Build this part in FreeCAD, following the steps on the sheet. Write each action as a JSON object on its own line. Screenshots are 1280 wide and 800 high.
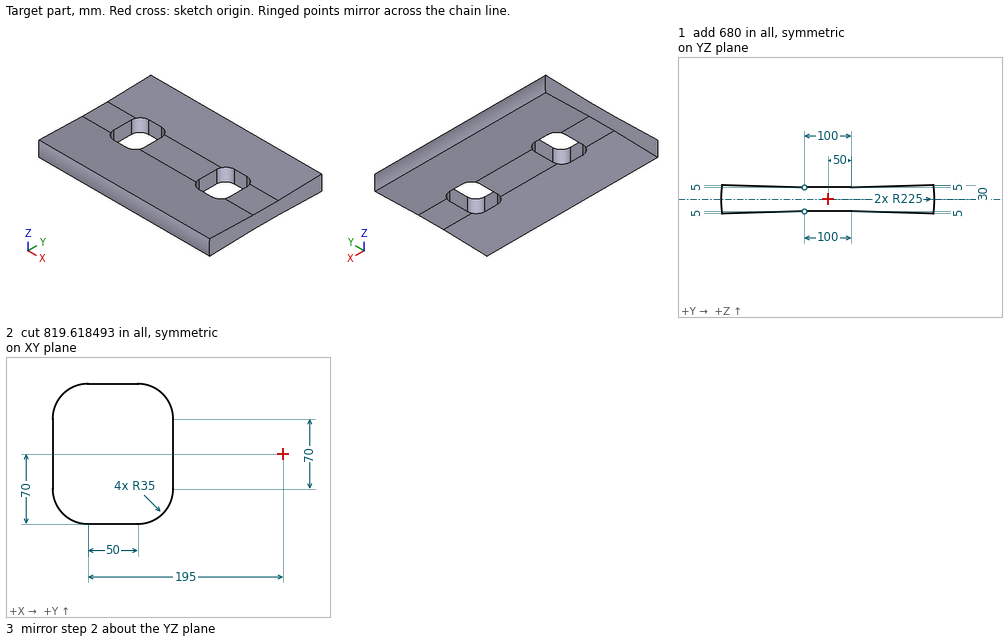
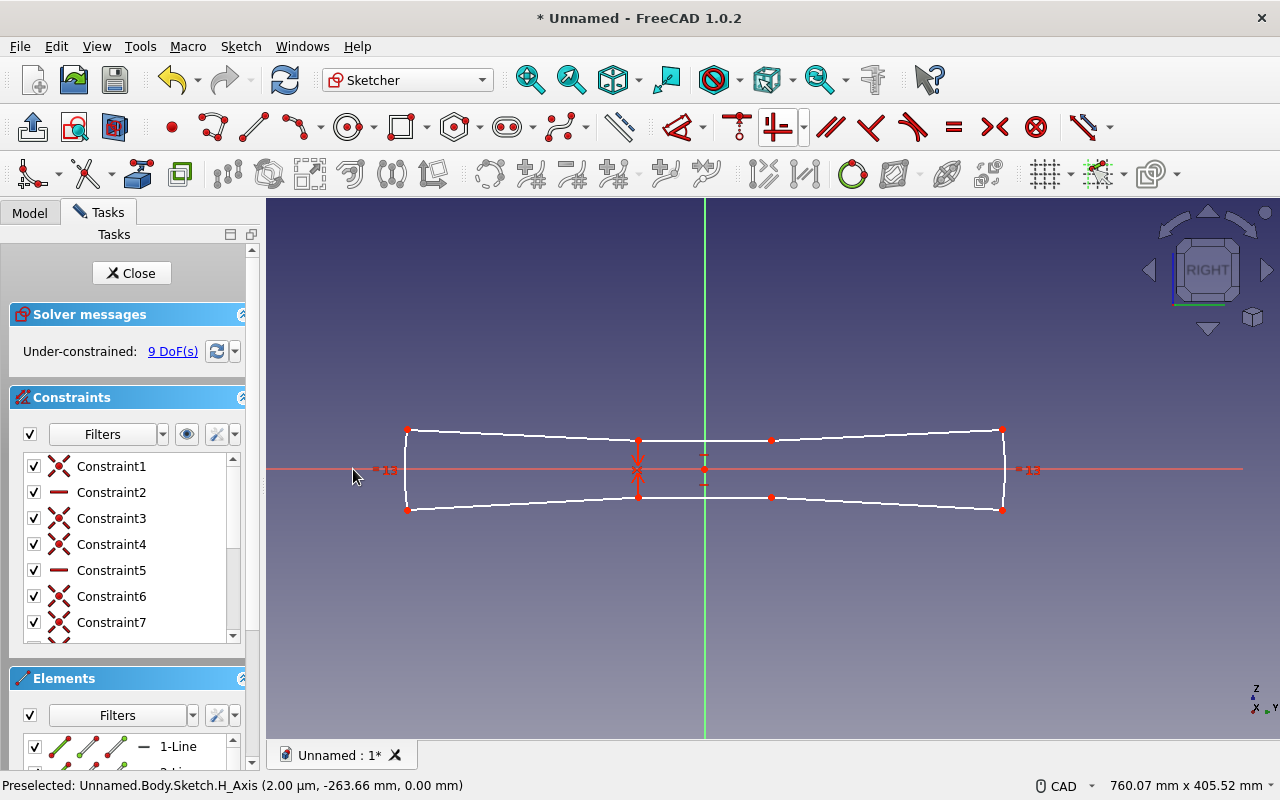
{"action": "left_click", "coordinate": [405, 454]}
{"action": "left_click", "coordinate": [373, 452]}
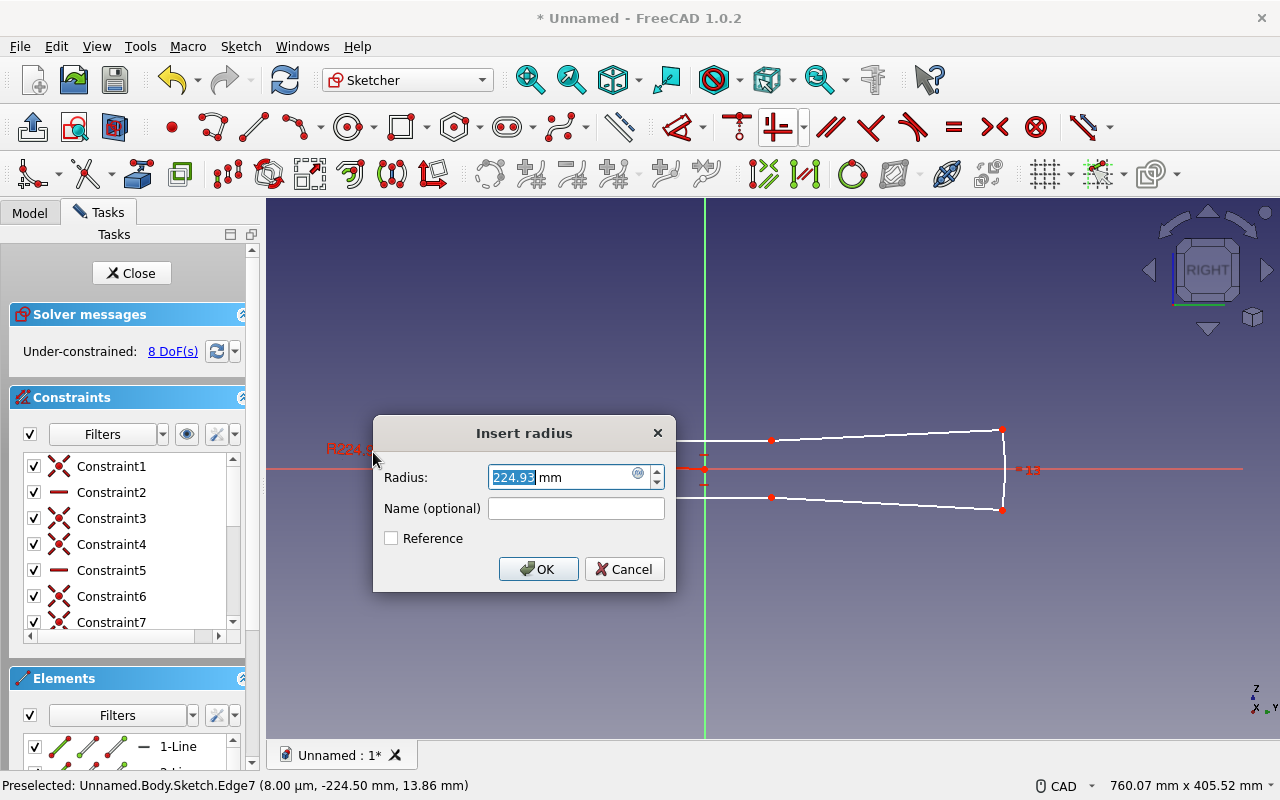
{"action": "type", "text": "225"}
{"action": "key", "text": "Return"}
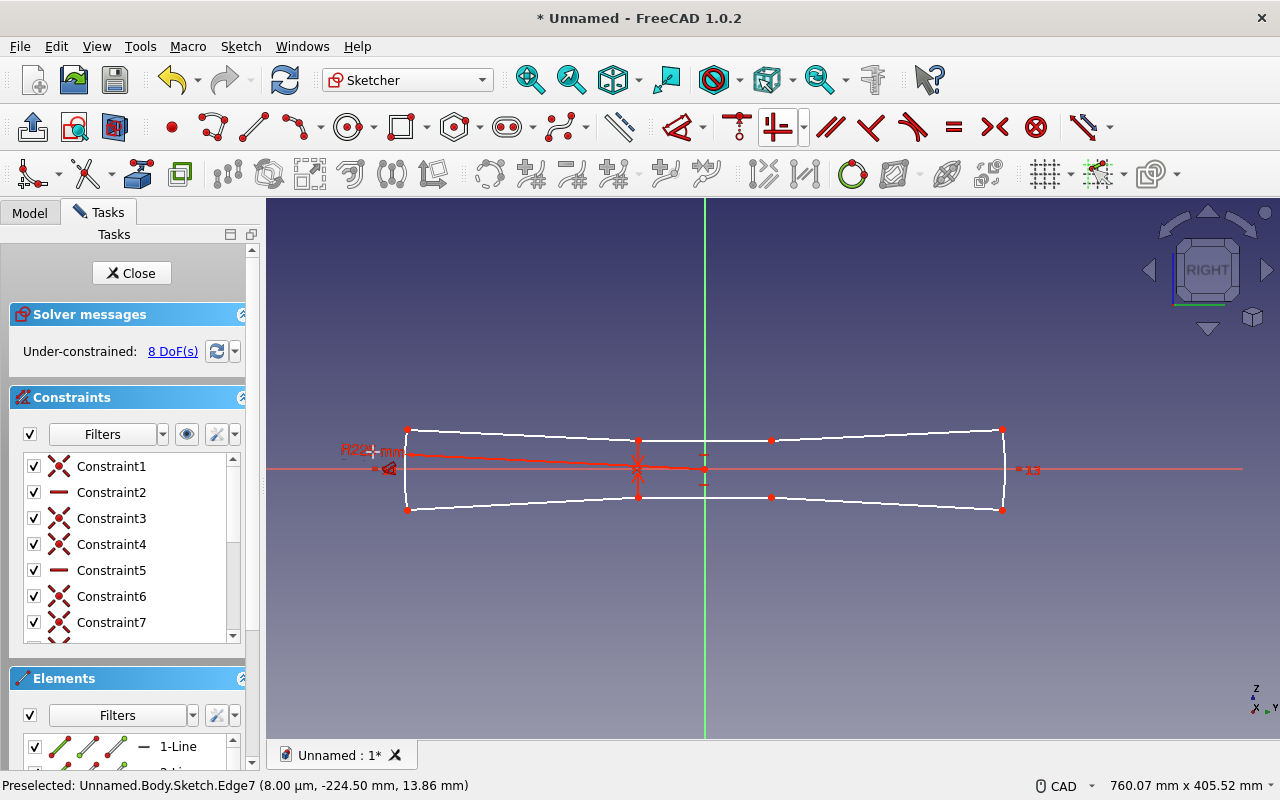
{"action": "scroll", "coordinate": [933, 433], "scroll_direction": "up", "scroll_amount": 9}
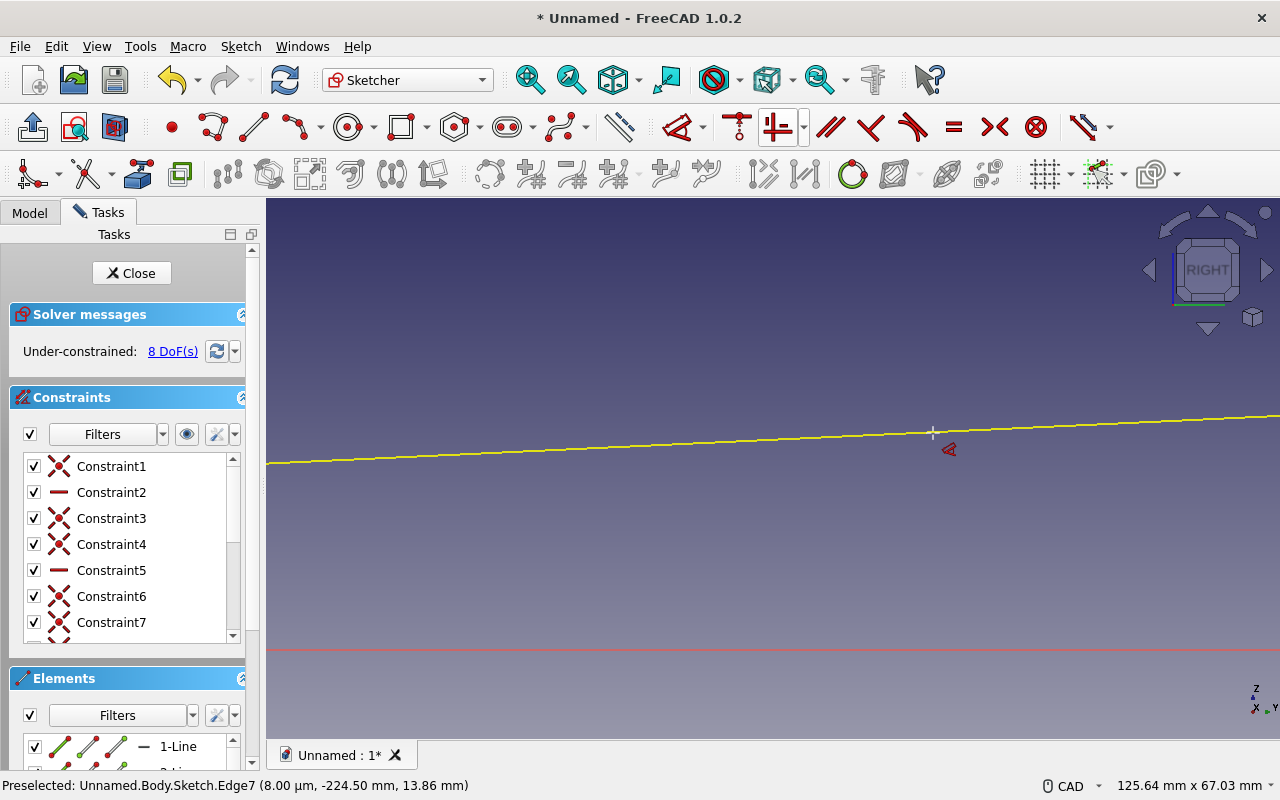
{"action": "left_click", "coordinate": [929, 432]}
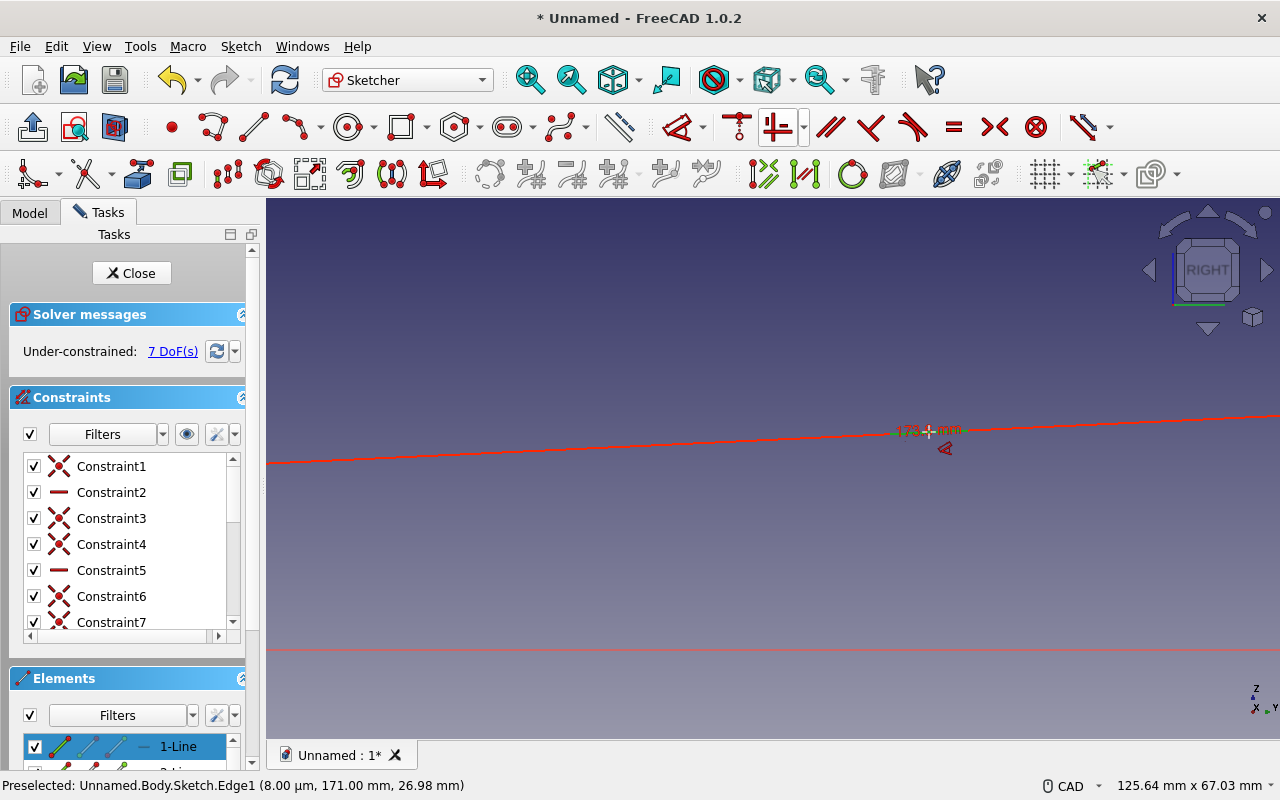
{"action": "key", "text": "Escape"}
{"action": "key", "text": "Escape"}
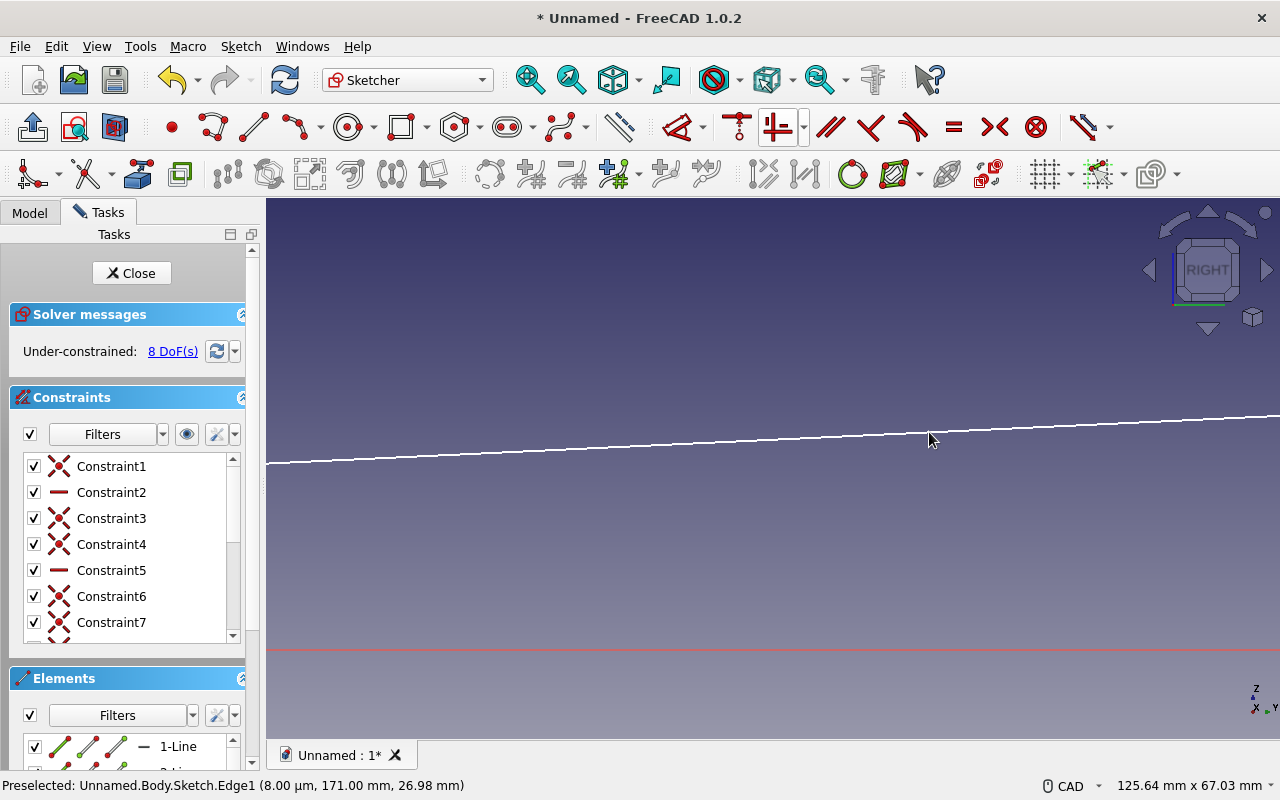
{"action": "left_click", "coordinate": [929, 432]}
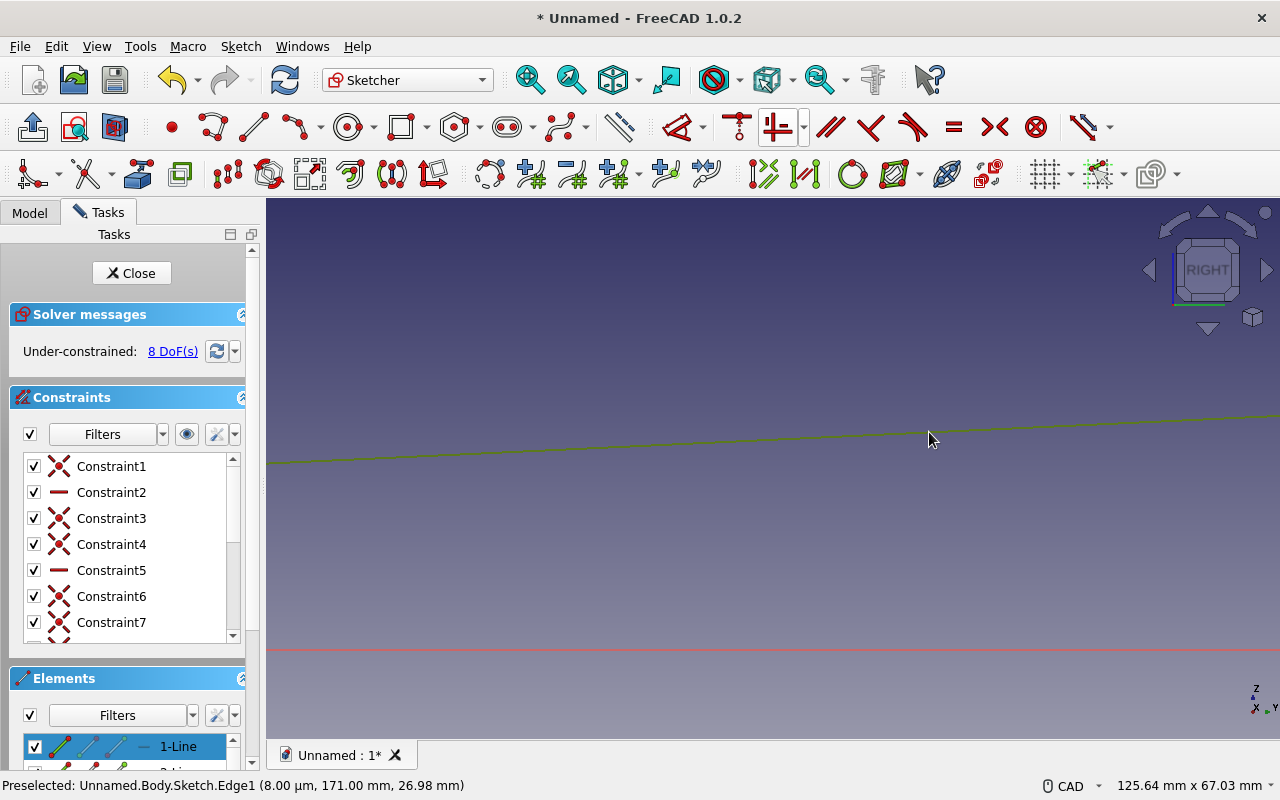
{"action": "key", "text": "i"}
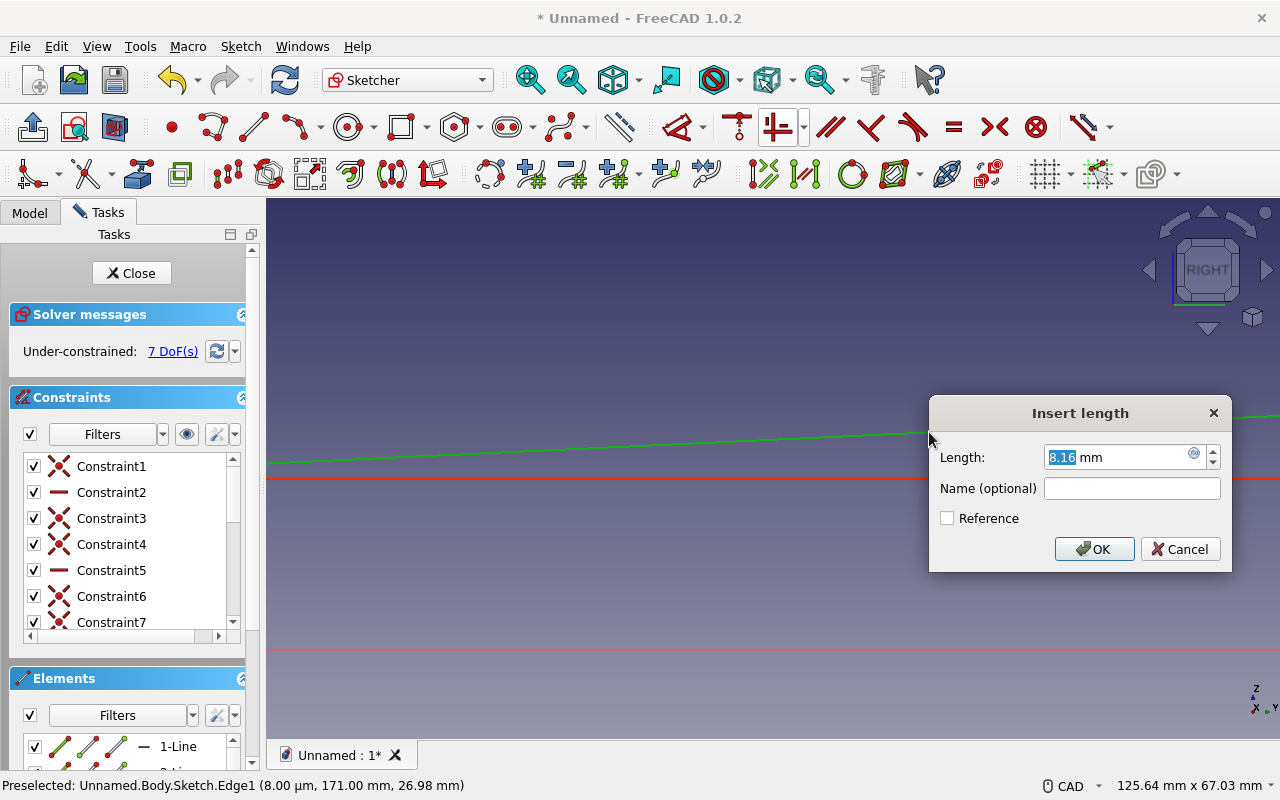
{"action": "type", "text": "5"}
{"action": "key", "text": "Return"}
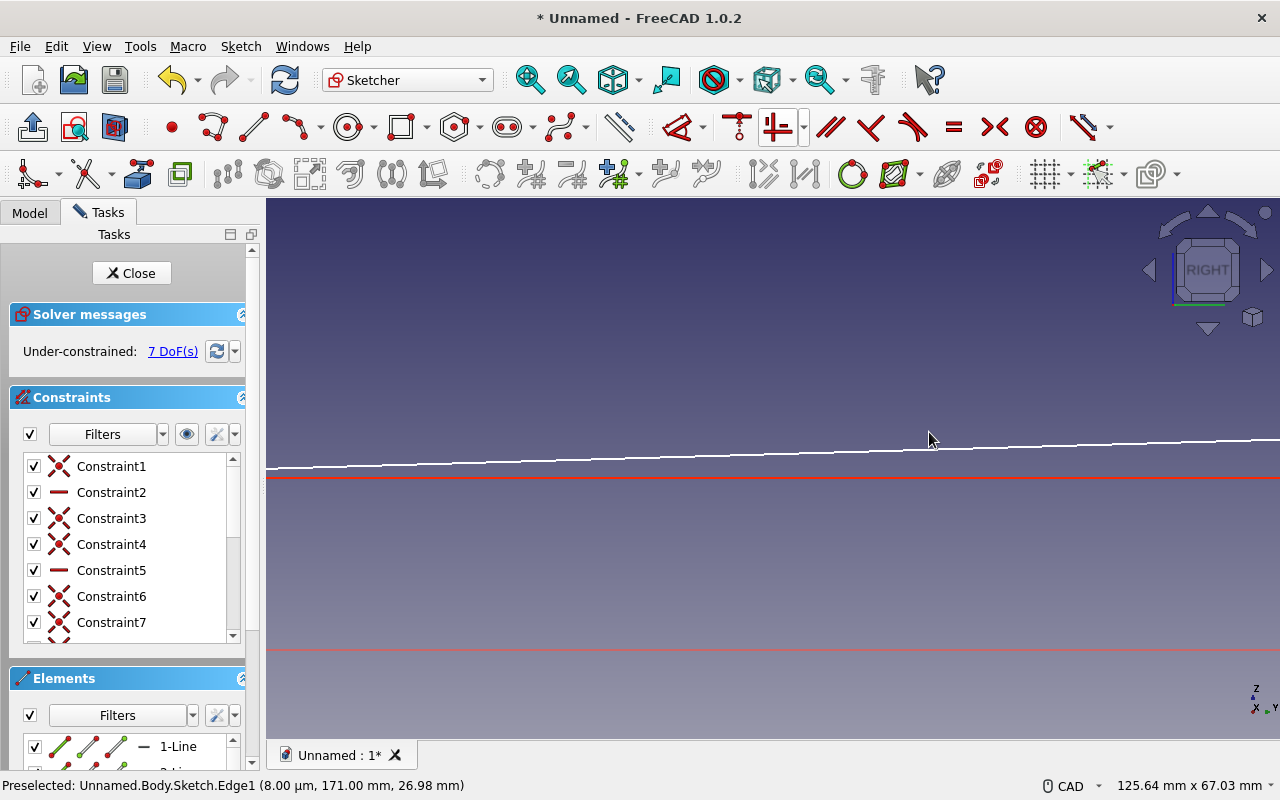
{"action": "scroll", "coordinate": [933, 433], "scroll_direction": "down", "scroll_amount": 9}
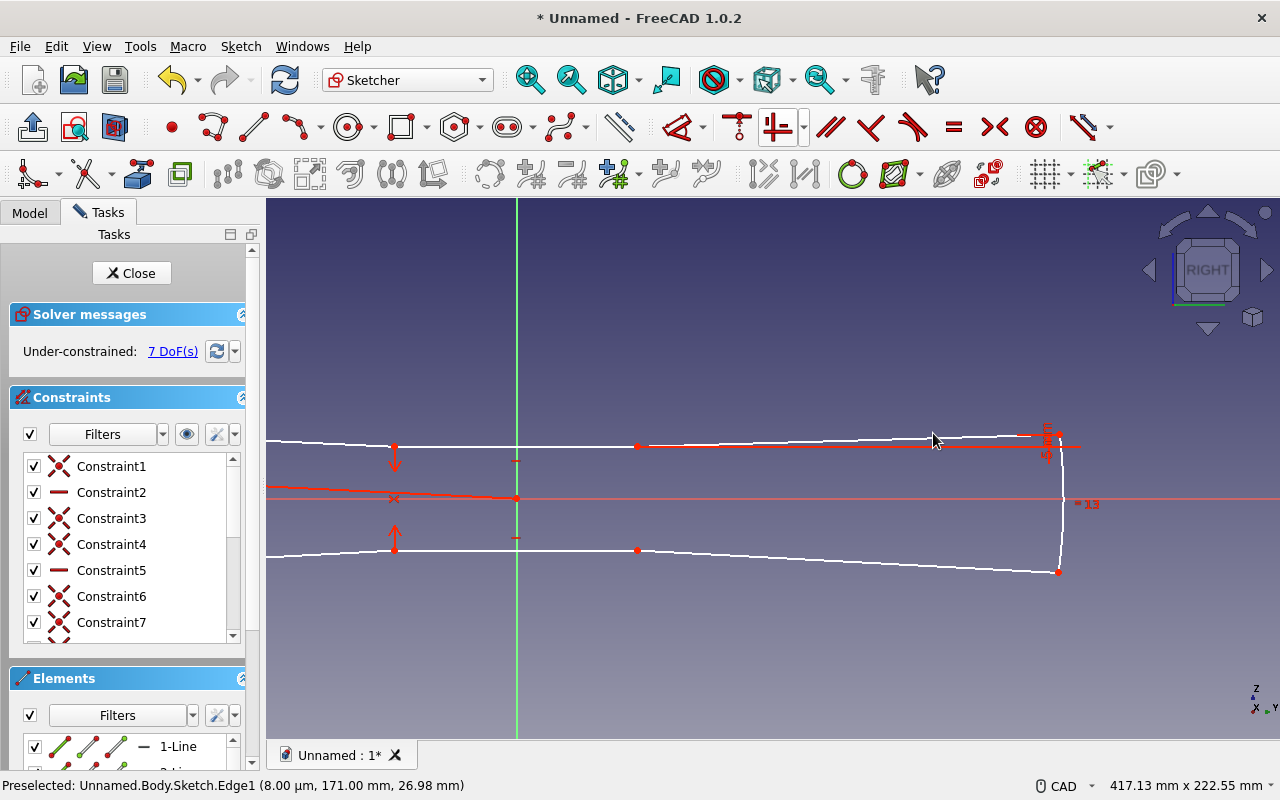
{"action": "scroll", "coordinate": [569, 438], "scroll_direction": "up", "scroll_amount": 9}